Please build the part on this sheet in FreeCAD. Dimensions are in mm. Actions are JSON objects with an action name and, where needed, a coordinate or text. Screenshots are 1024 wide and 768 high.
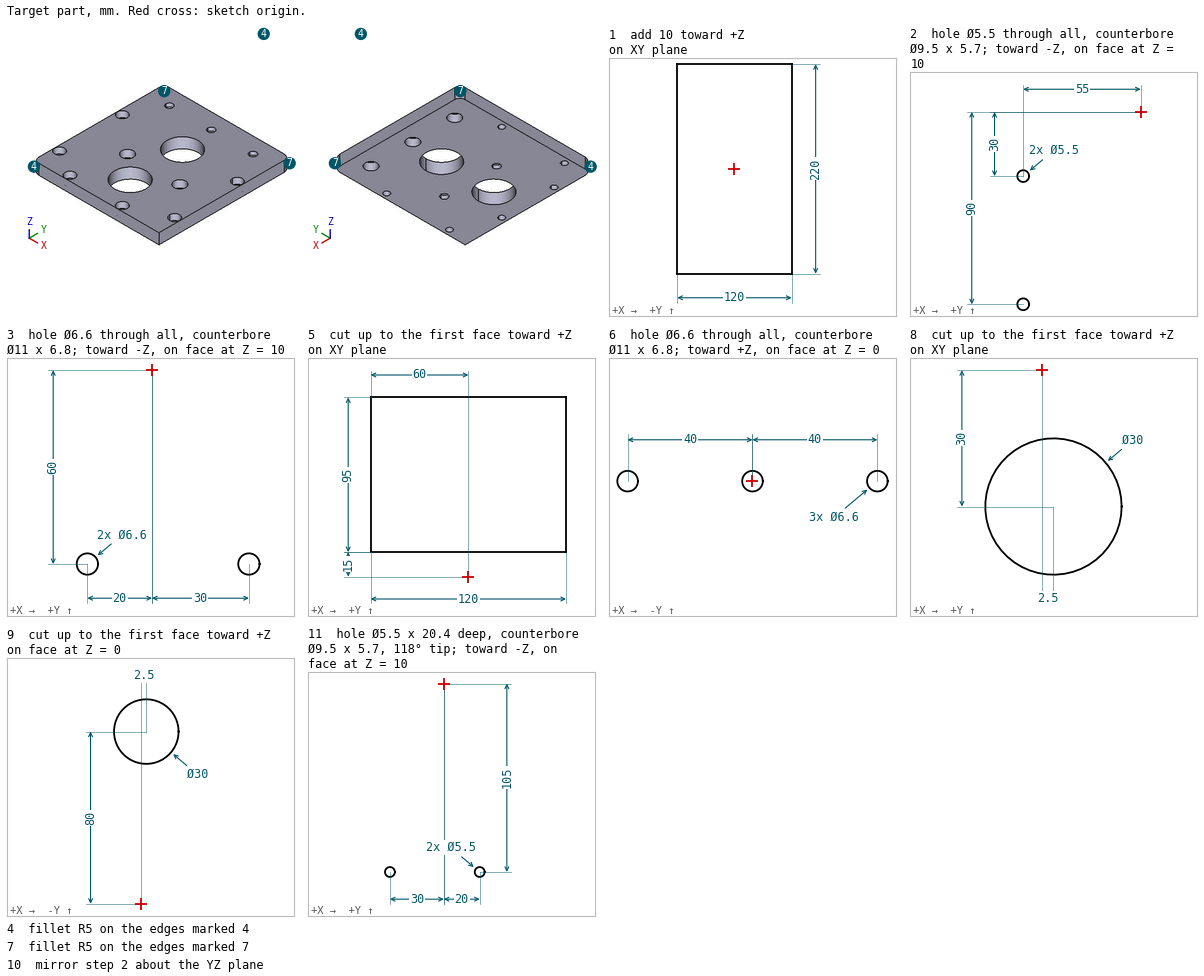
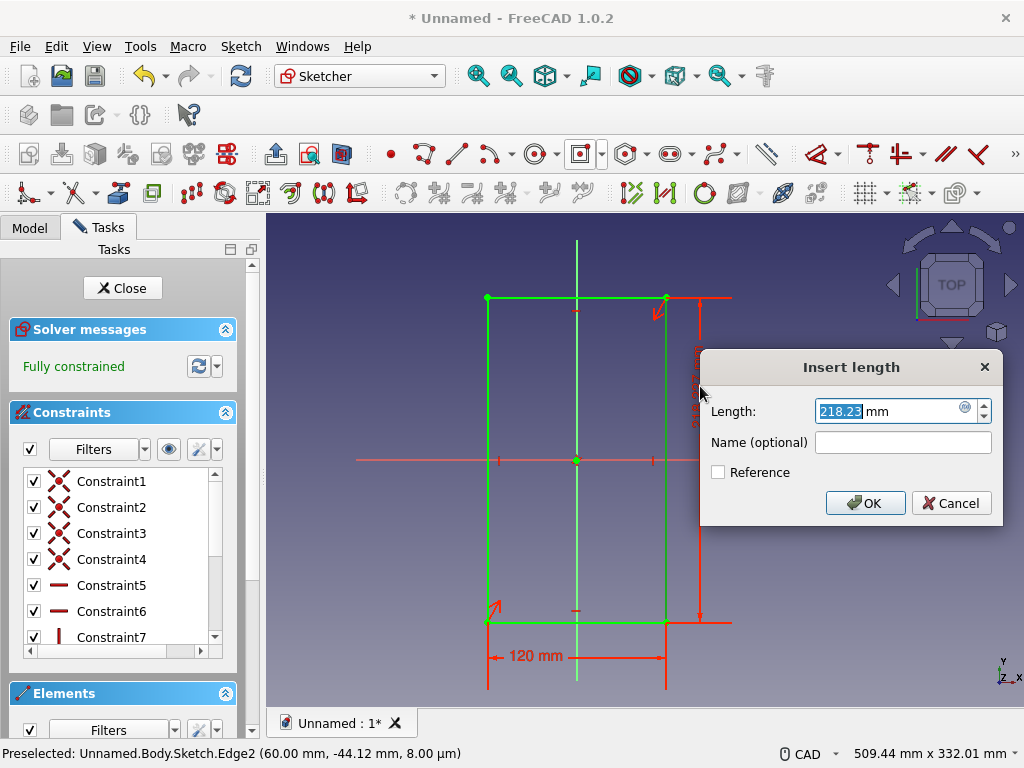
{"action": "type", "text": "220"}
{"action": "key", "text": "Return"}
{"action": "key", "text": "Escape"}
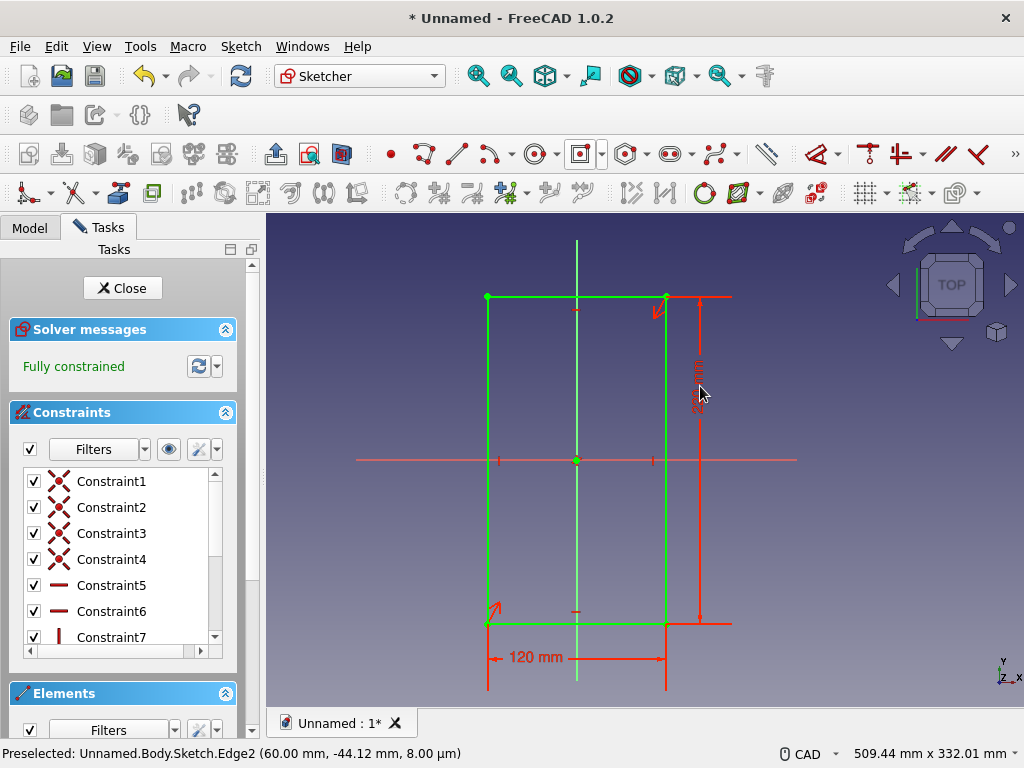
{"action": "left_click", "coordinate": [123, 288]}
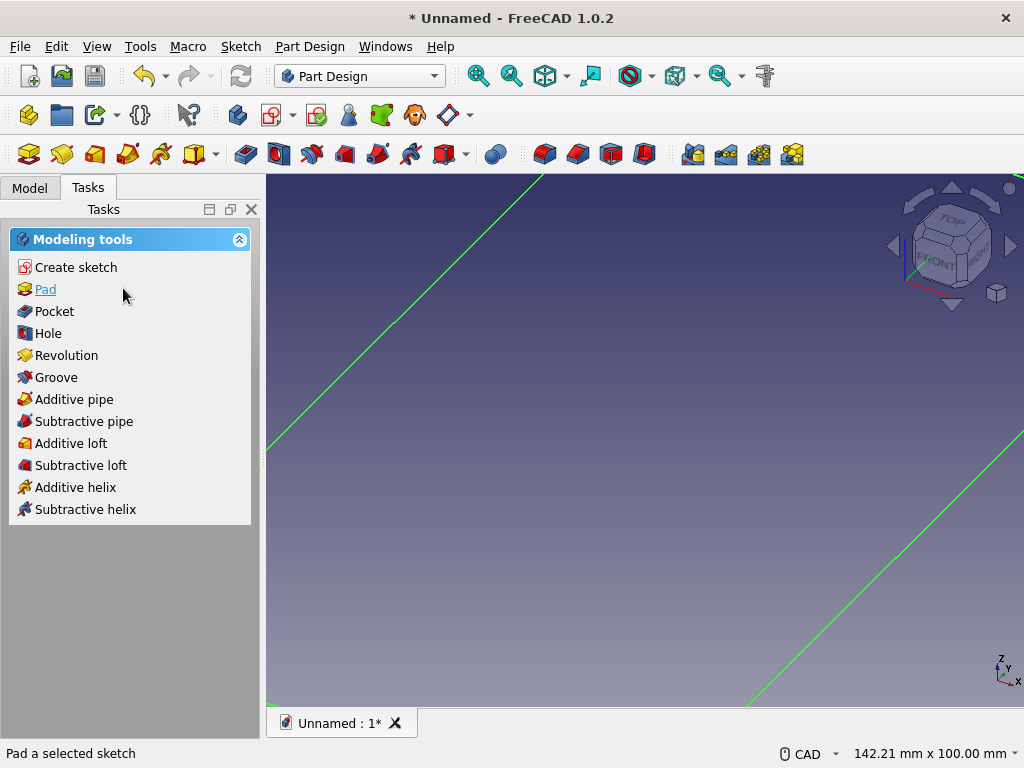
{"action": "left_click", "coordinate": [29, 154]}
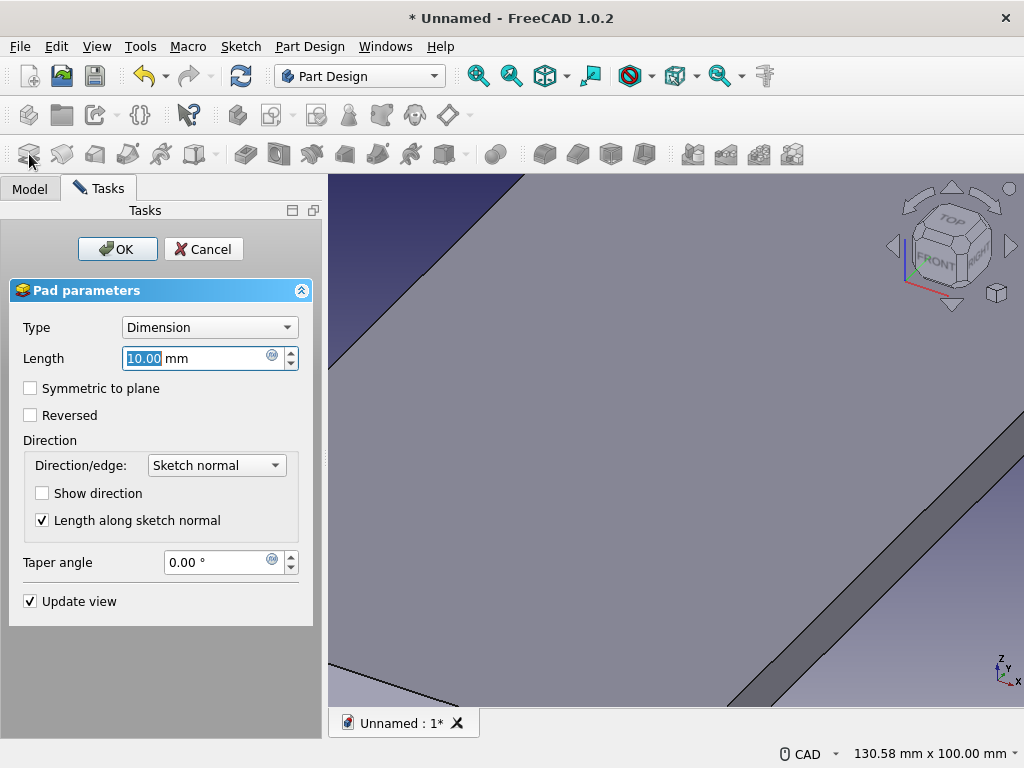
{"action": "type", "text": "10"}
{"action": "key", "text": "Tab"}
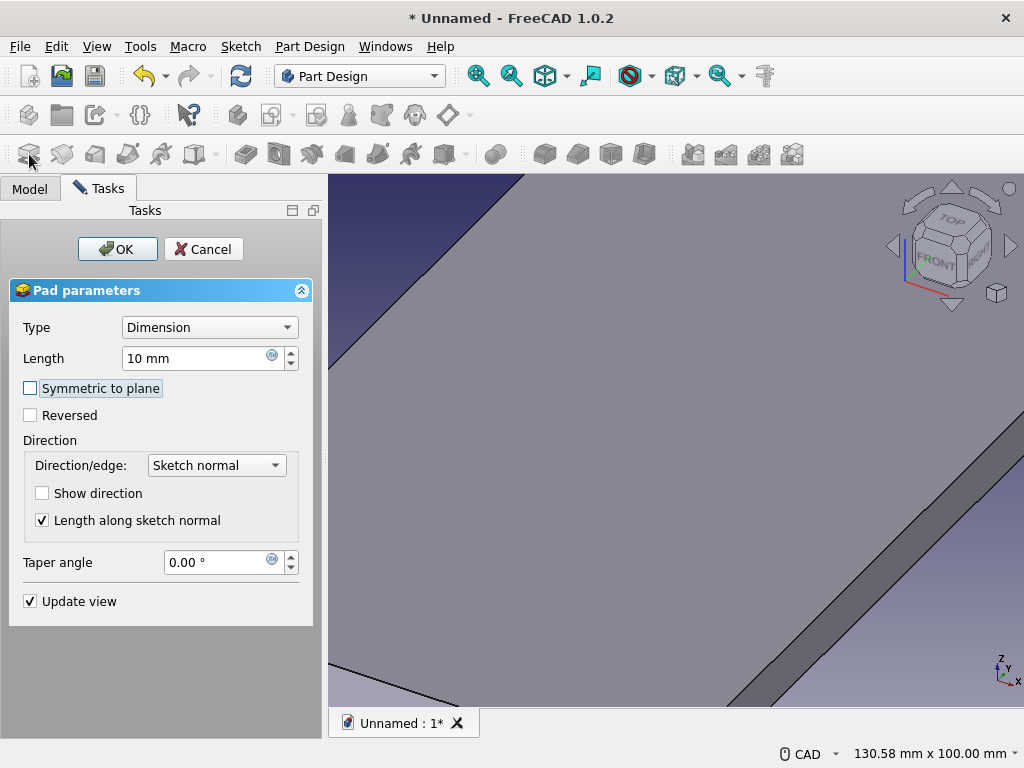
{"action": "left_click", "coordinate": [118, 249]}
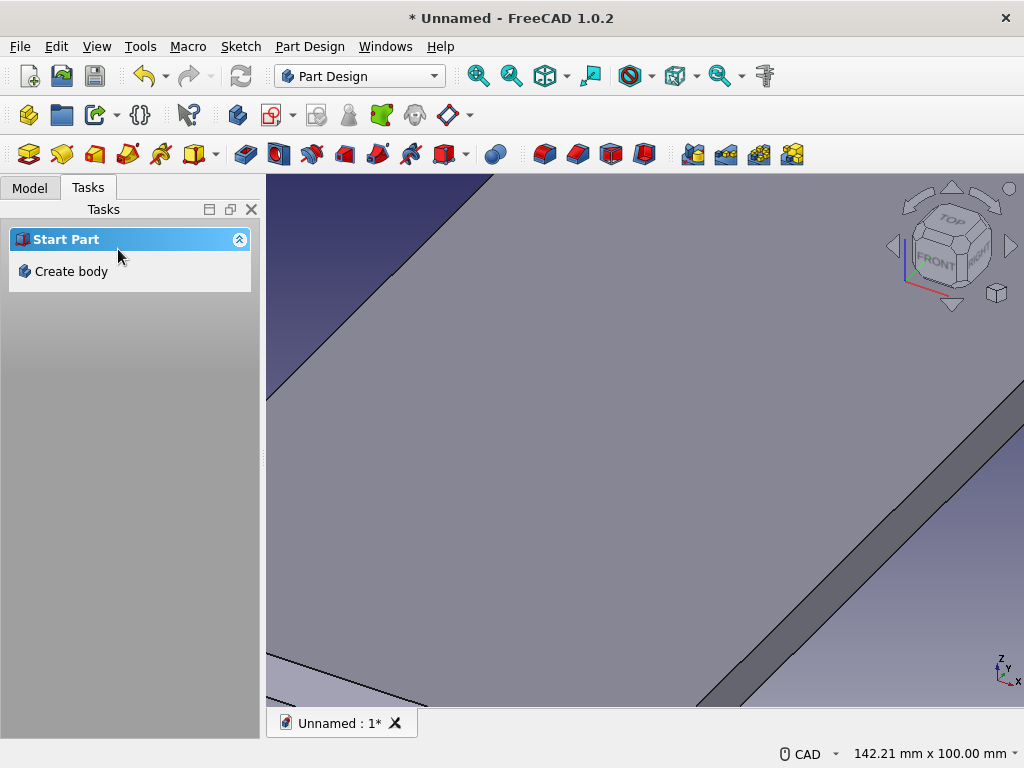
{"action": "left_click", "coordinate": [479, 76]}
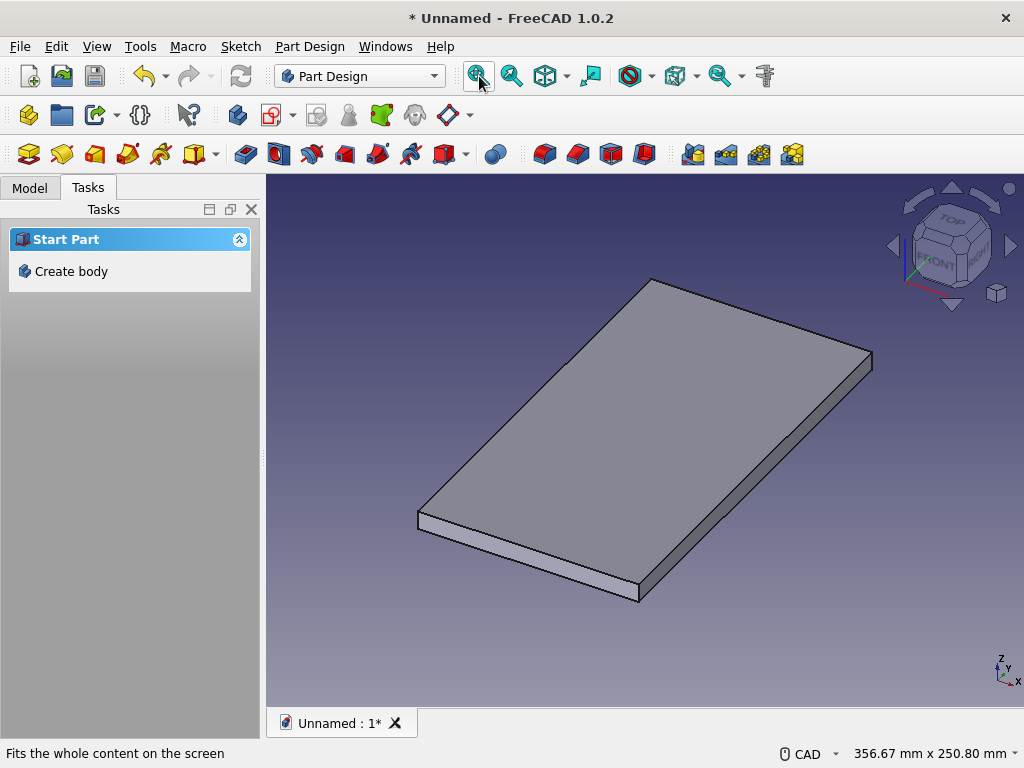
{"action": "left_click", "coordinate": [678, 398]}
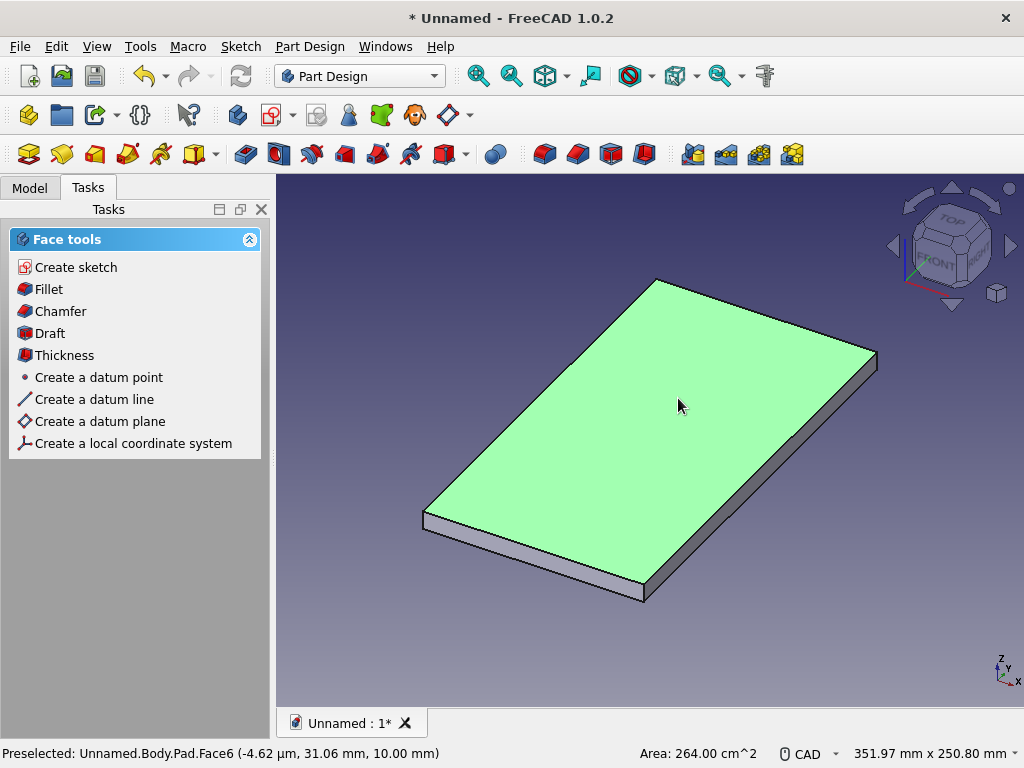
{"action": "left_click", "coordinate": [270, 116]}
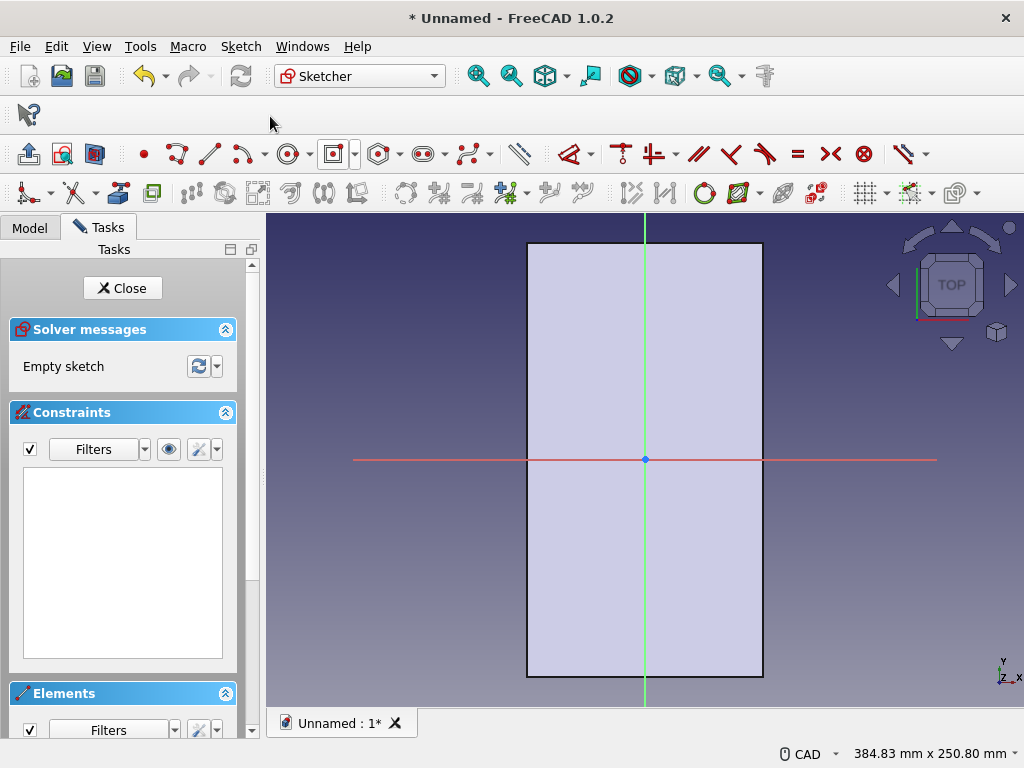
{"action": "scroll", "coordinate": [602, 662], "scroll_direction": "up", "scroll_amount": 3}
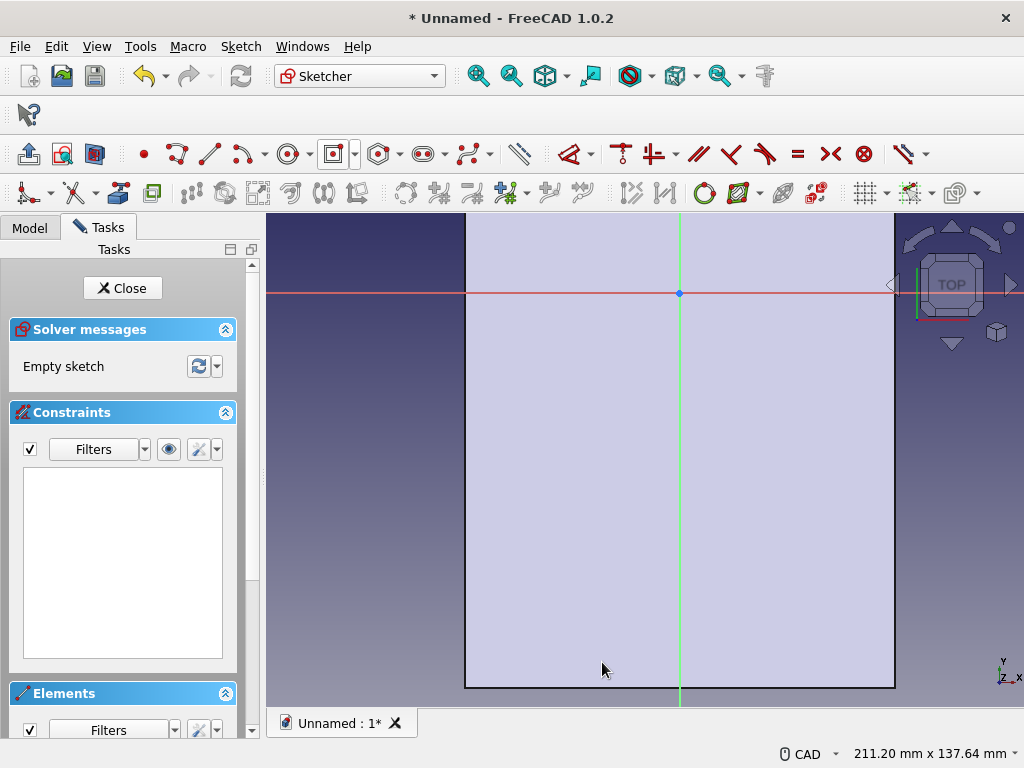
{"action": "left_click", "coordinate": [288, 154]}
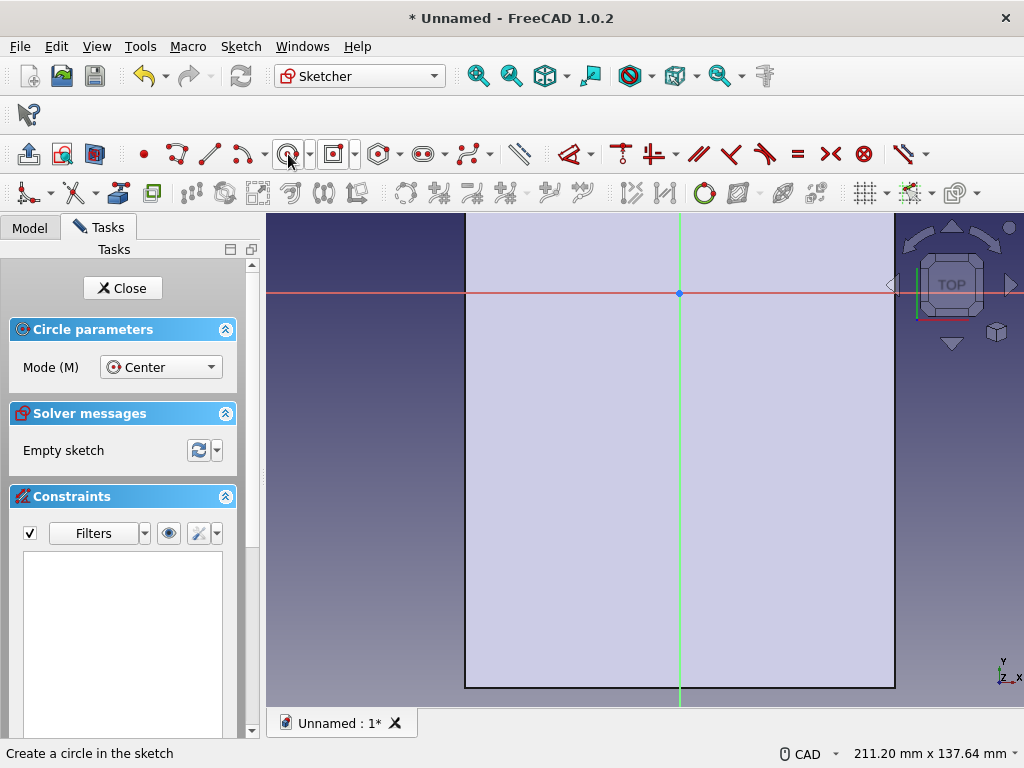
{"action": "scroll", "coordinate": [483, 401], "scroll_direction": "up", "scroll_amount": 5}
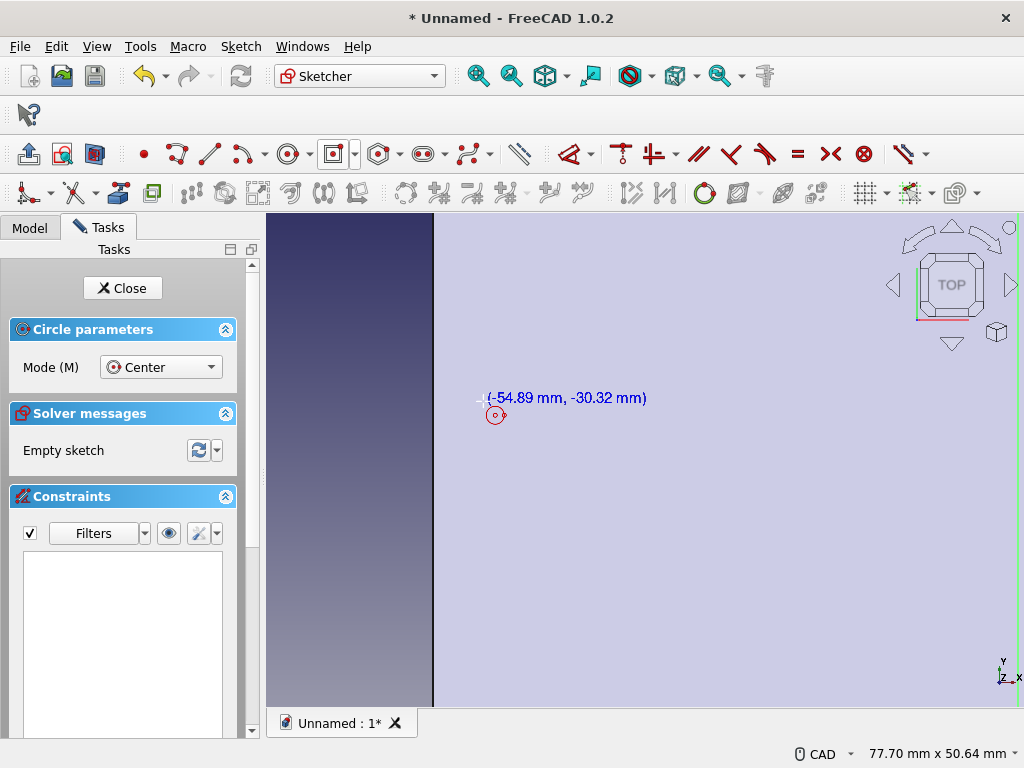
{"action": "left_click", "coordinate": [481, 400]}
{"action": "left_click", "coordinate": [500, 381]}